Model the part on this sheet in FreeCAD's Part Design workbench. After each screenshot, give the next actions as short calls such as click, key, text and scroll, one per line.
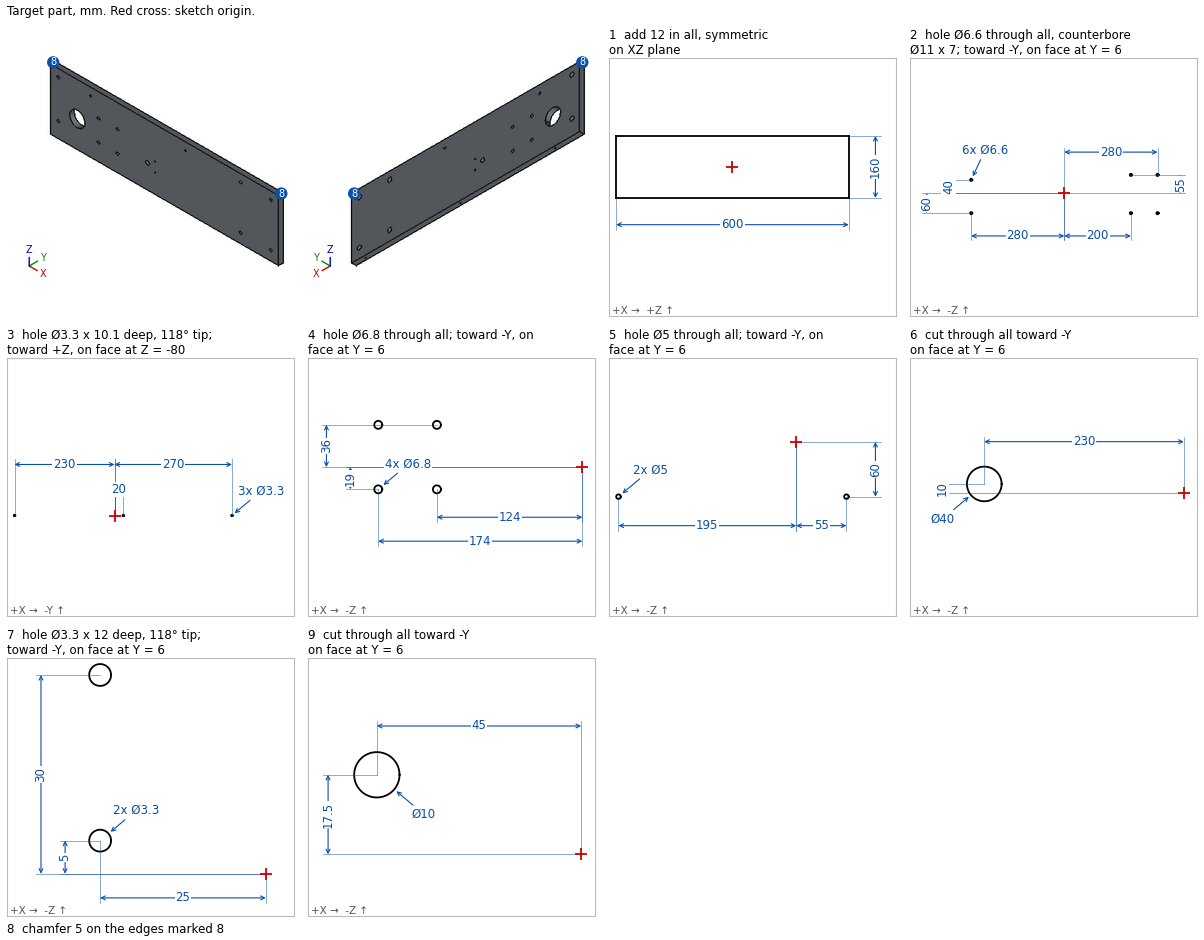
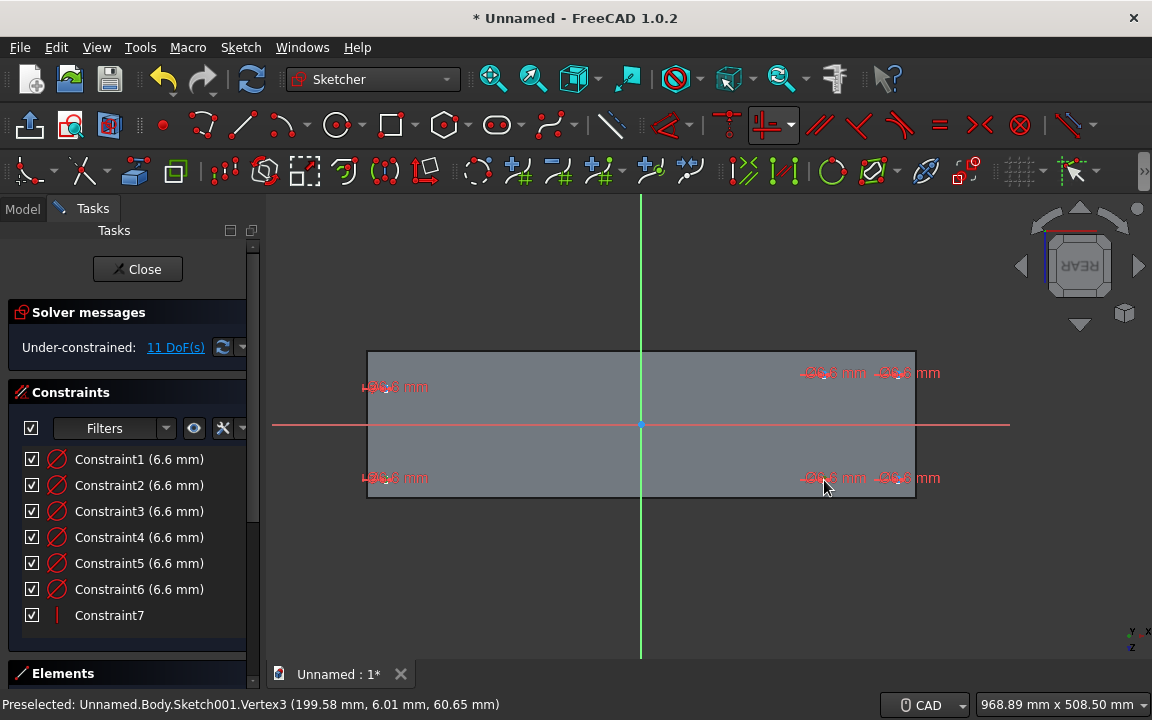
click(794, 126)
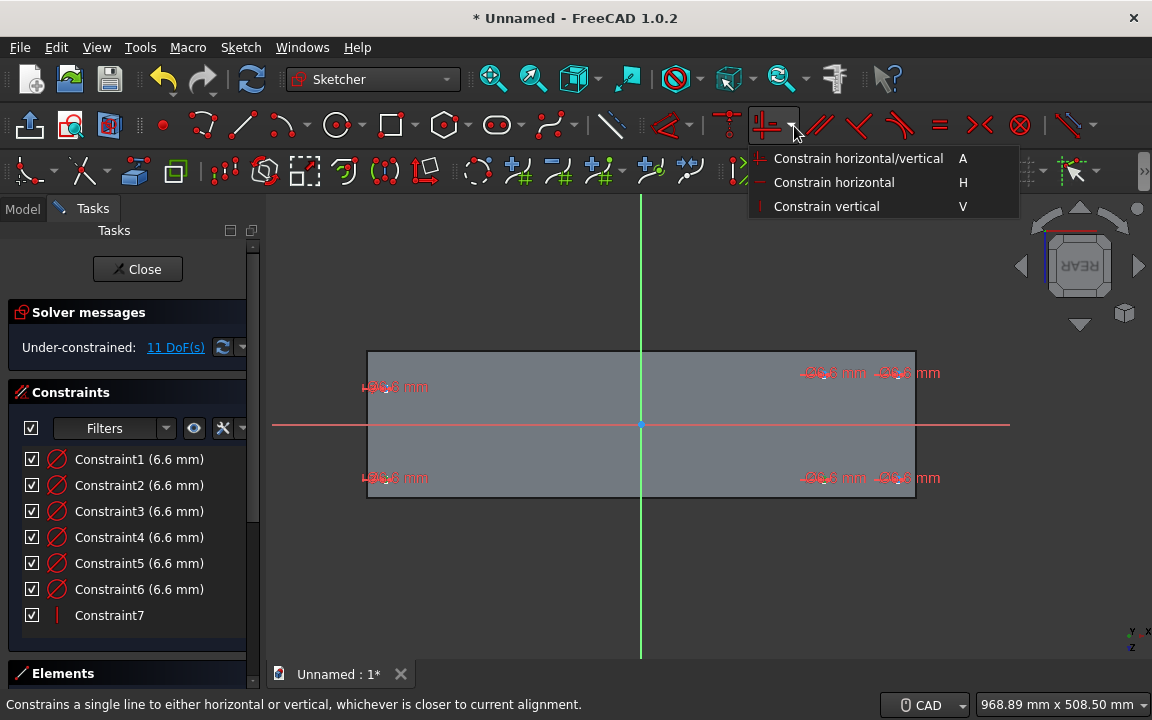
click(884, 182)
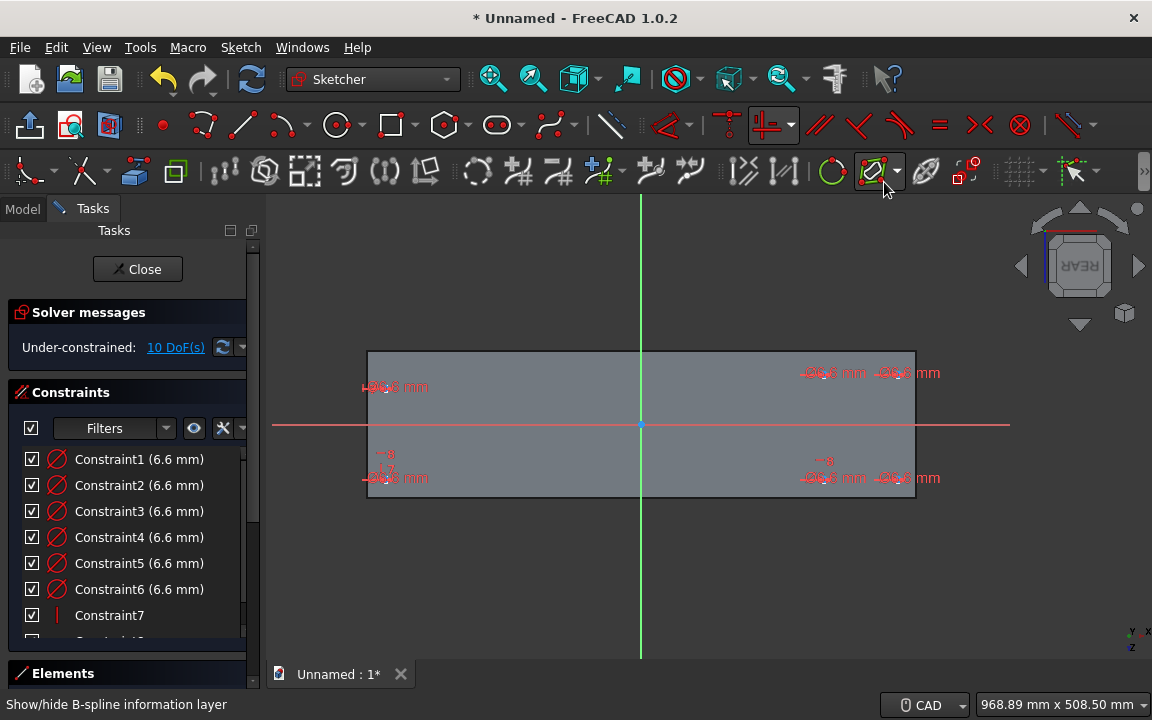
click(824, 480)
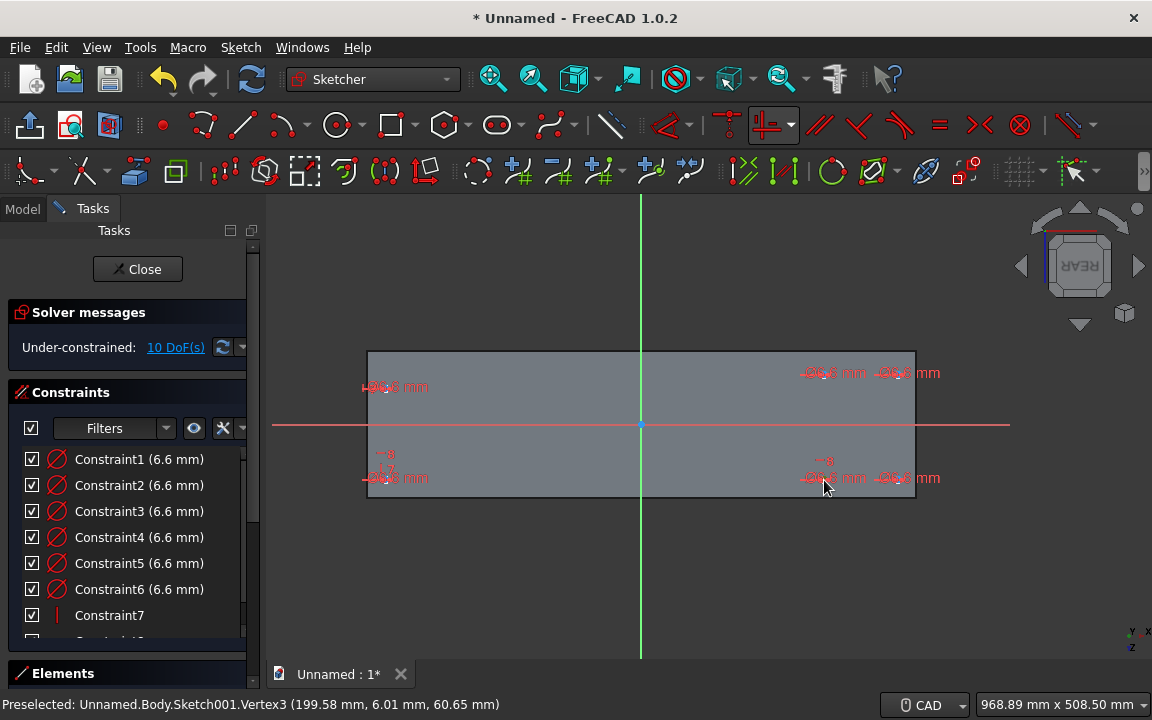
click(824, 375)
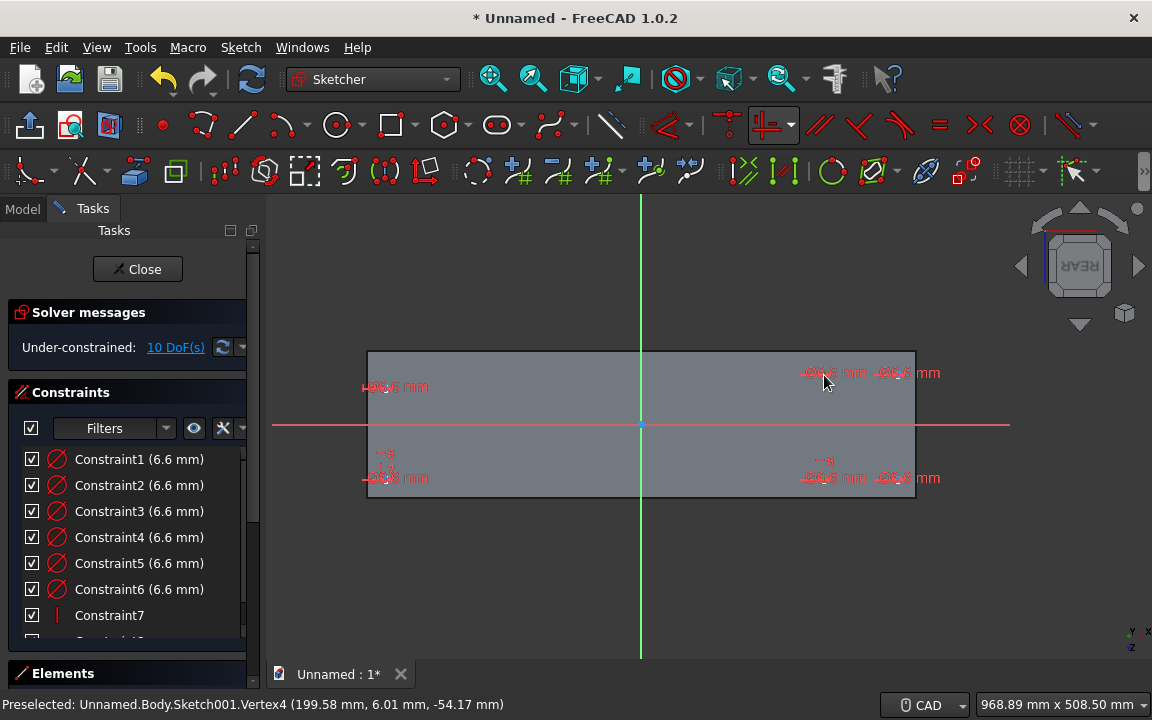
key(v)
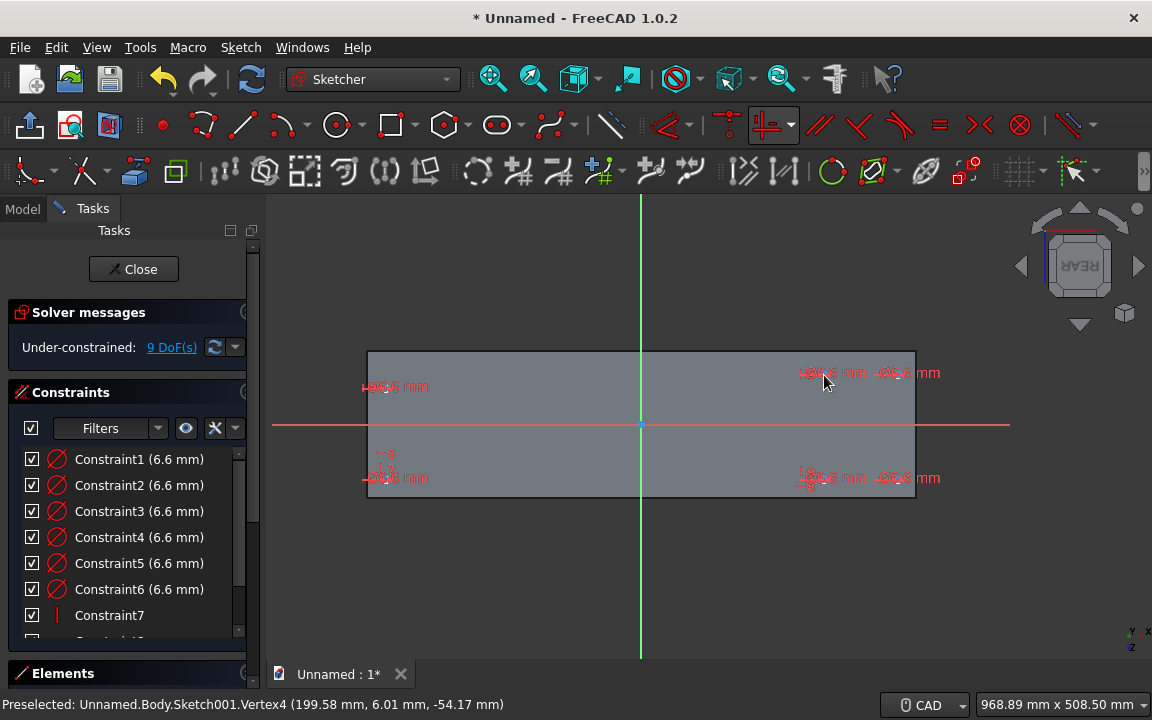
click(824, 375)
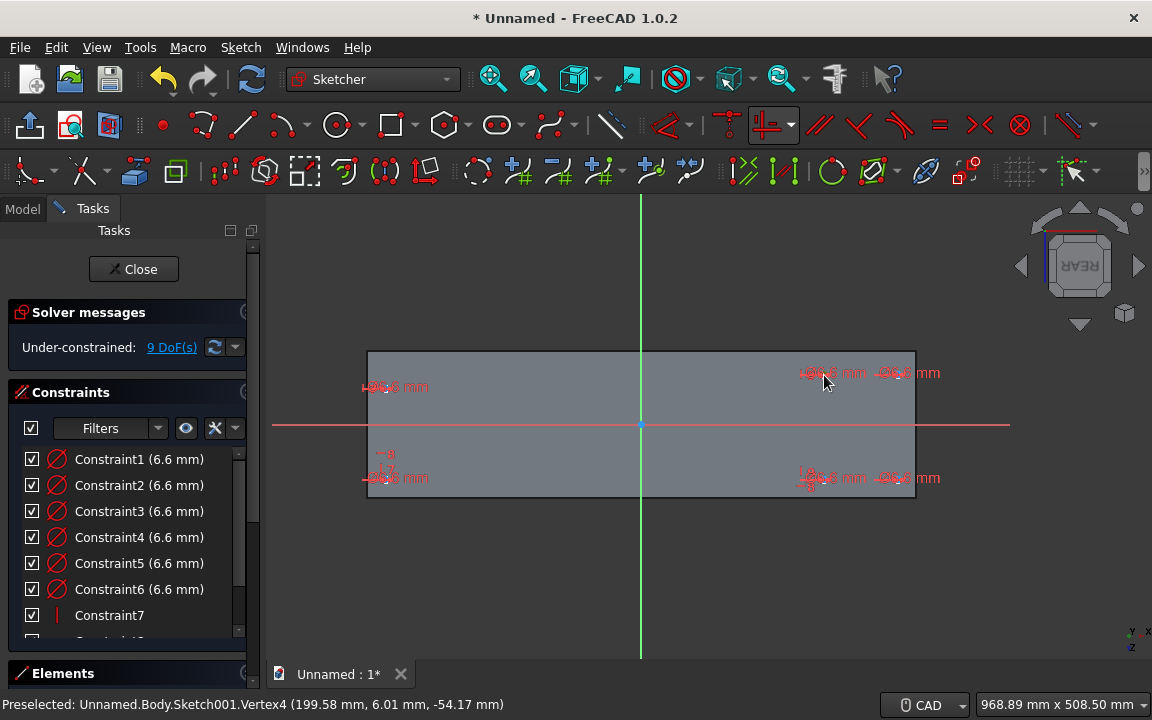
click(898, 375)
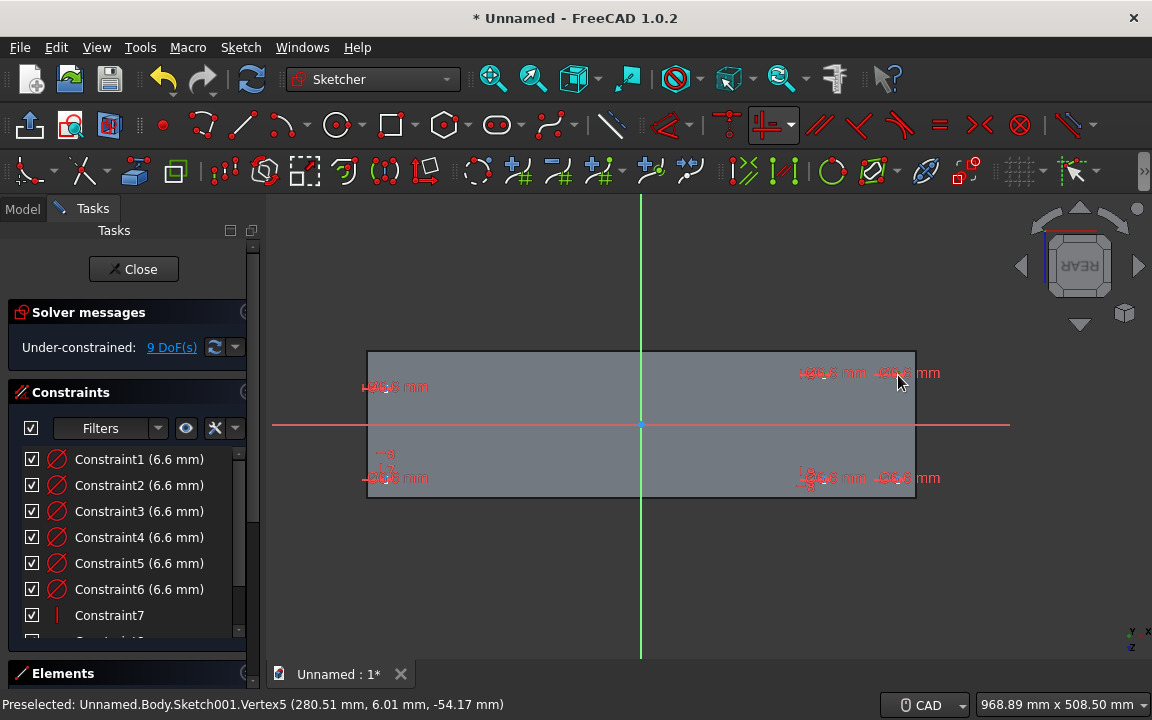
click(794, 126)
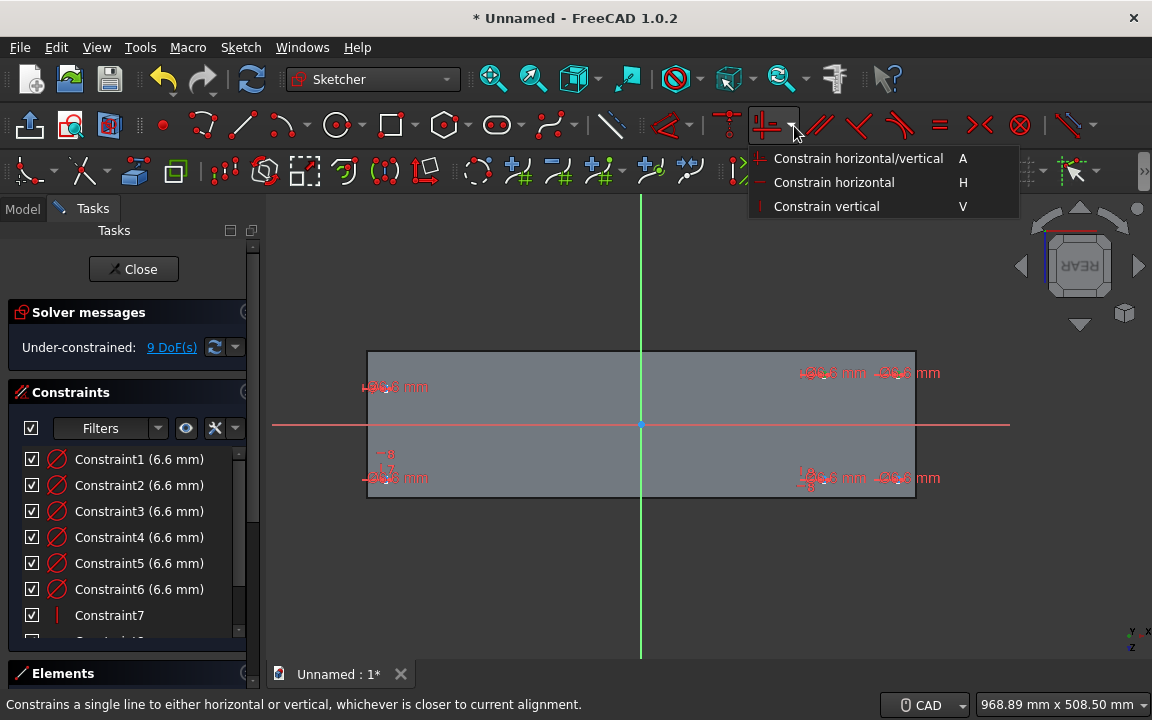
click(884, 182)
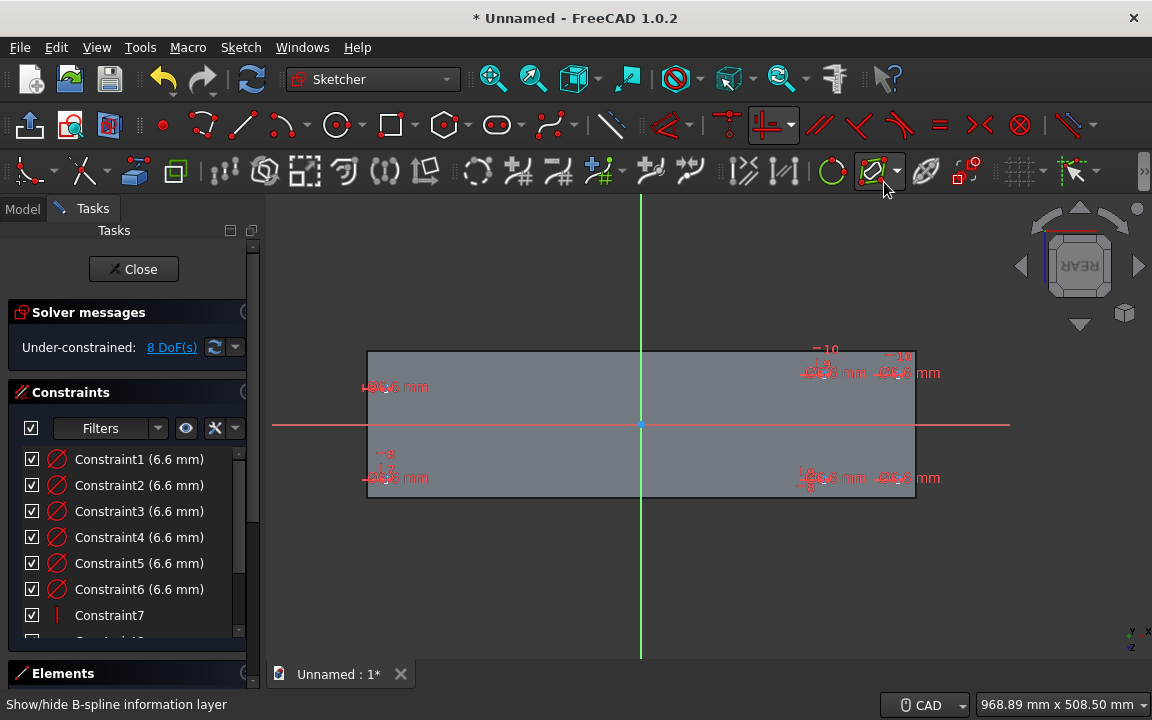
click(898, 375)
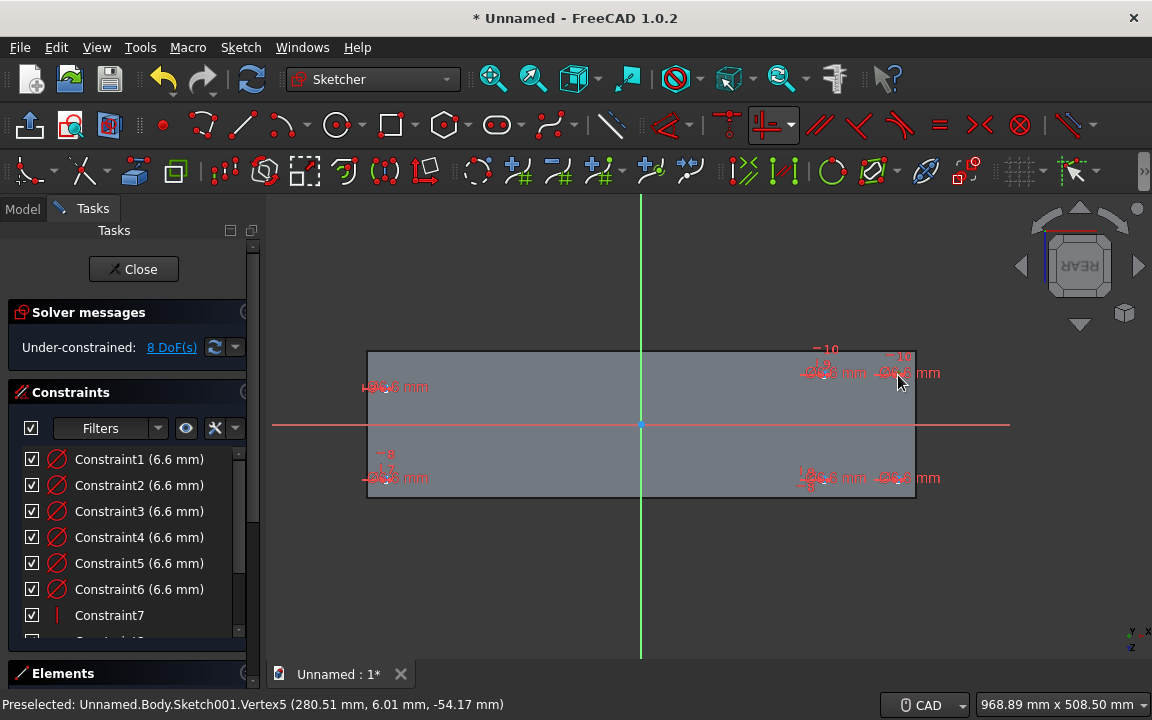
click(898, 480)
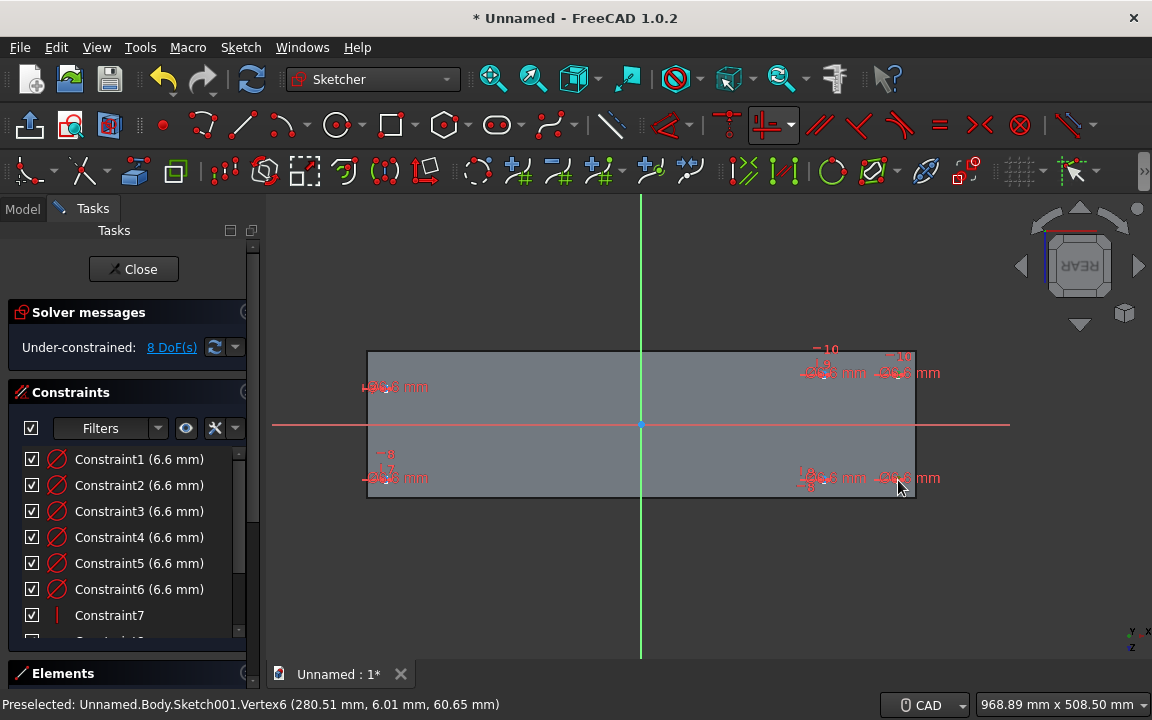
key(v)